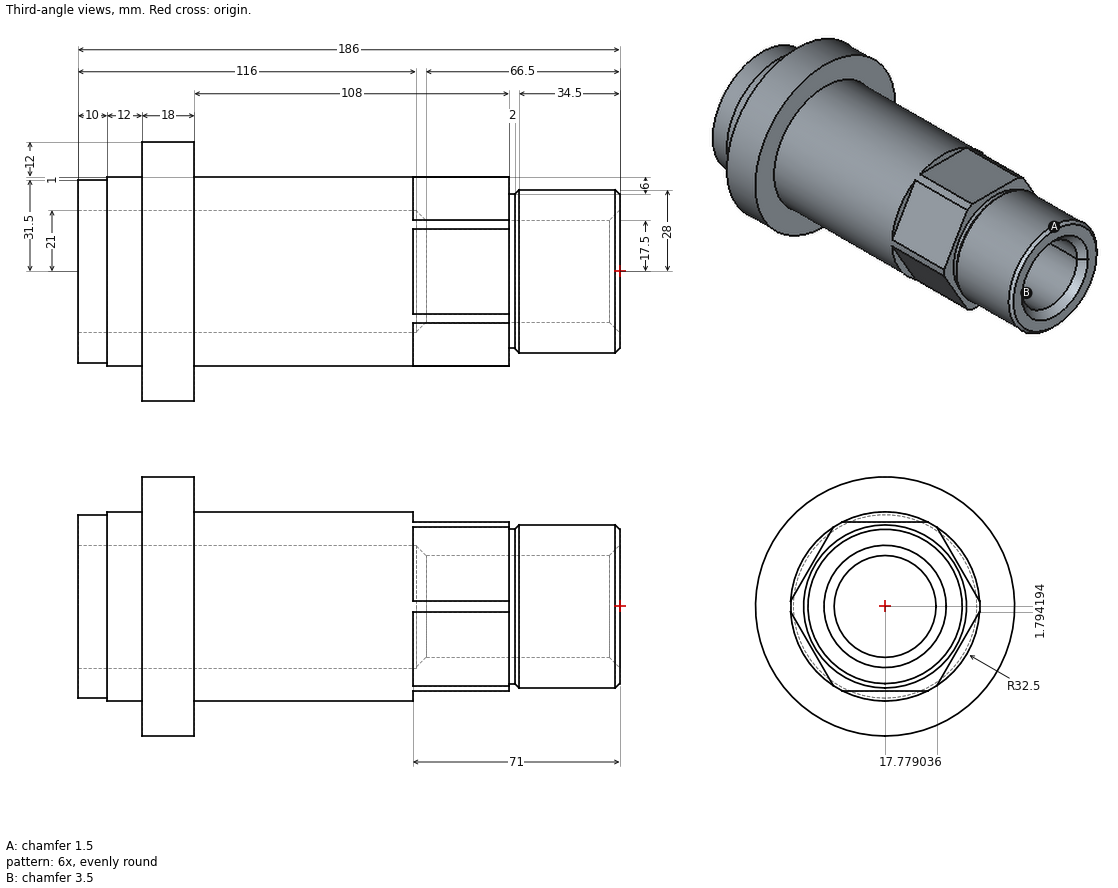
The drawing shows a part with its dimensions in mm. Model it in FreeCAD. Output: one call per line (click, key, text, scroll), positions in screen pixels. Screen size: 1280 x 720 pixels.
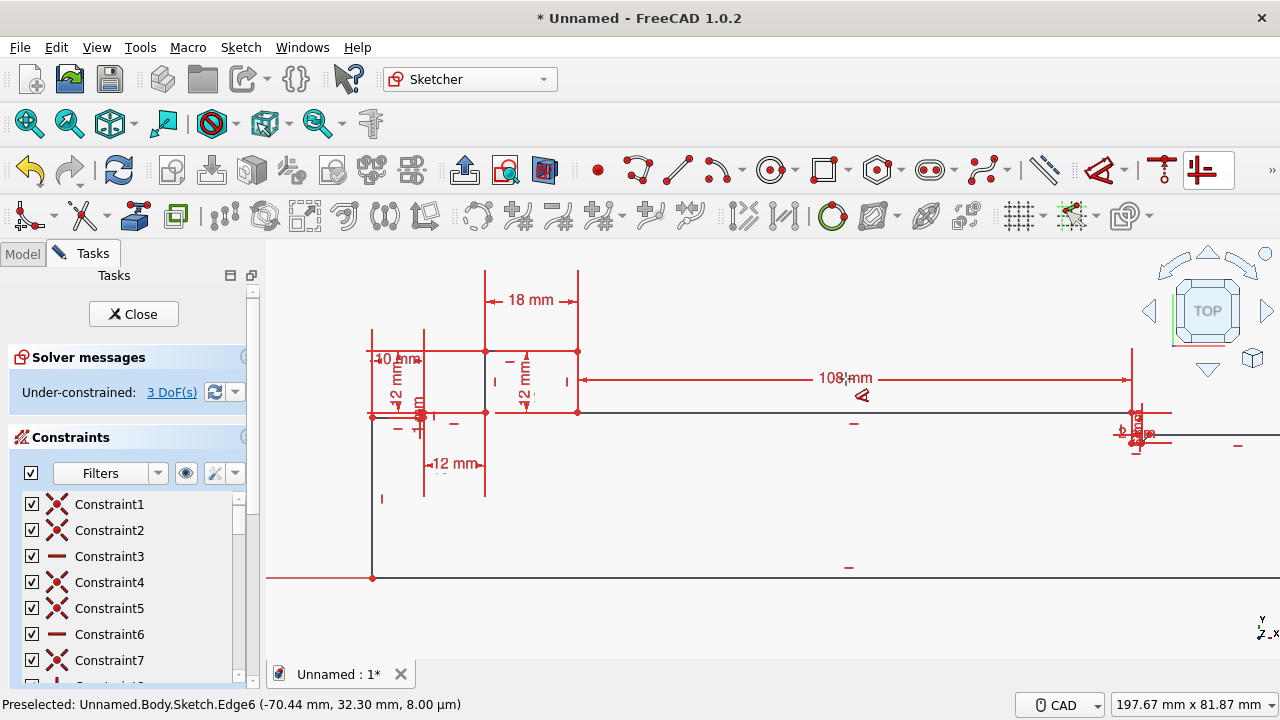
click(659, 578)
click(744, 612)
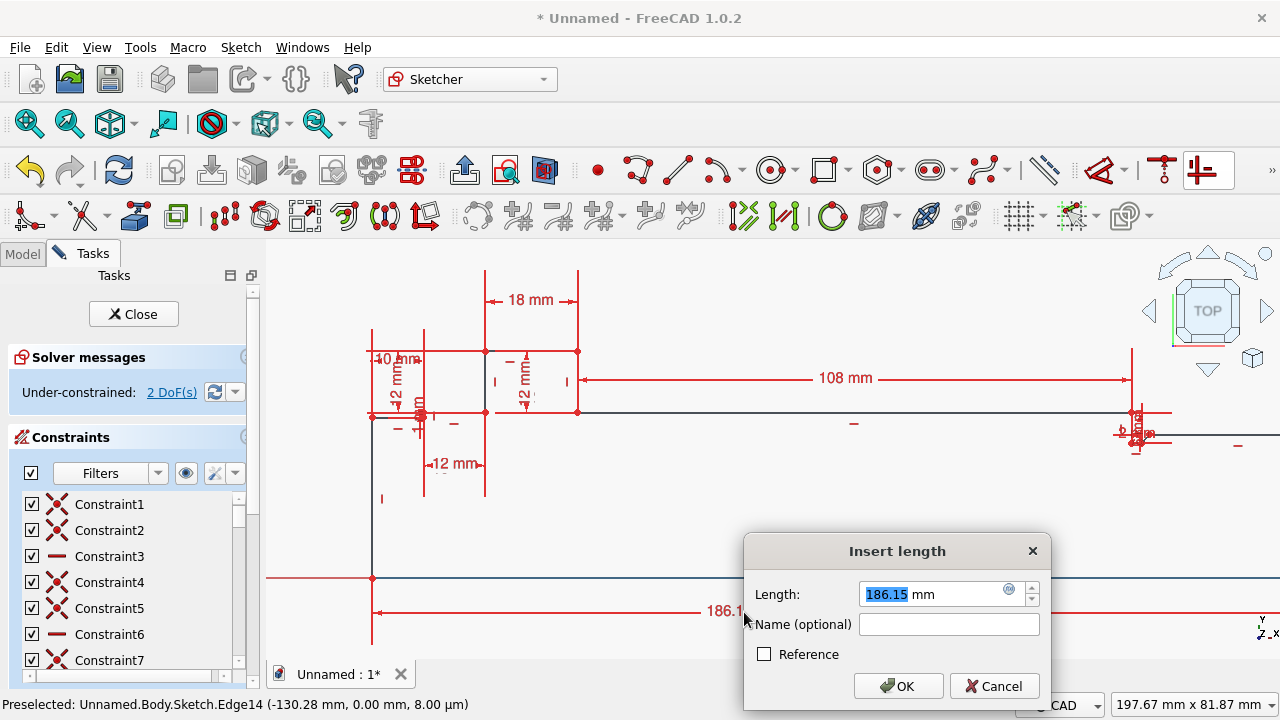
text(186)
key(Return)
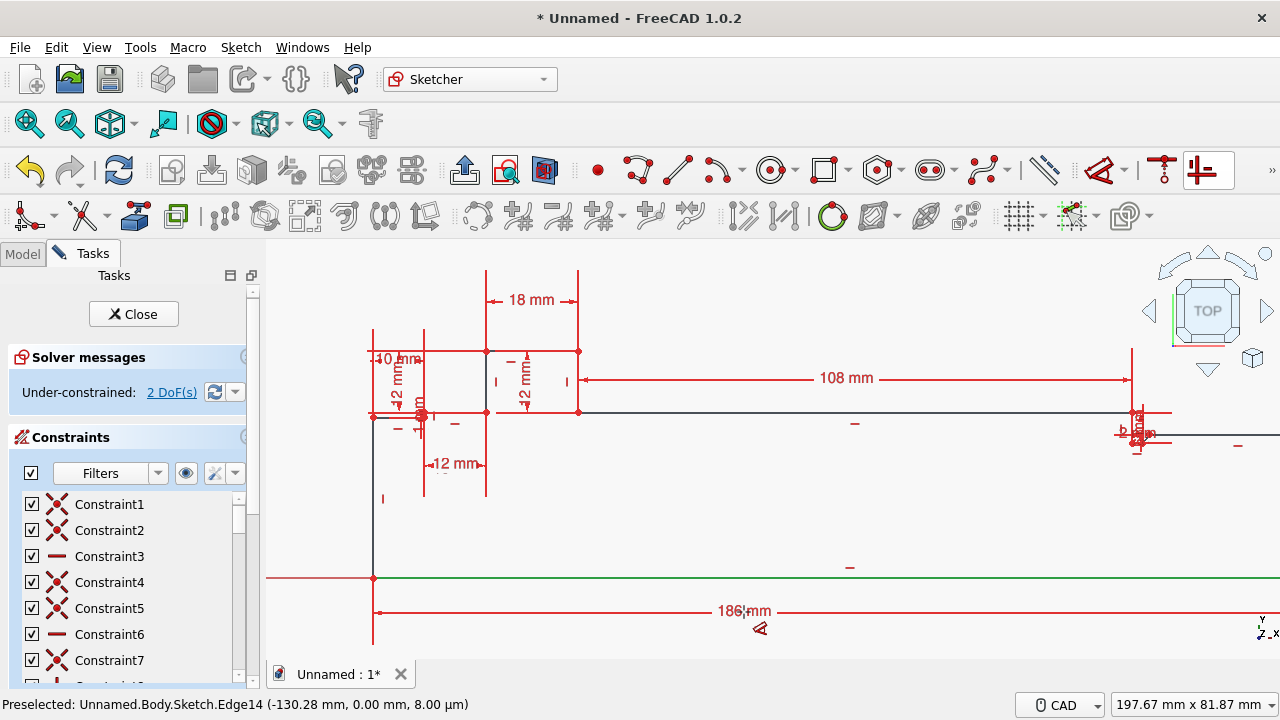
scroll(408, 418, down, 2)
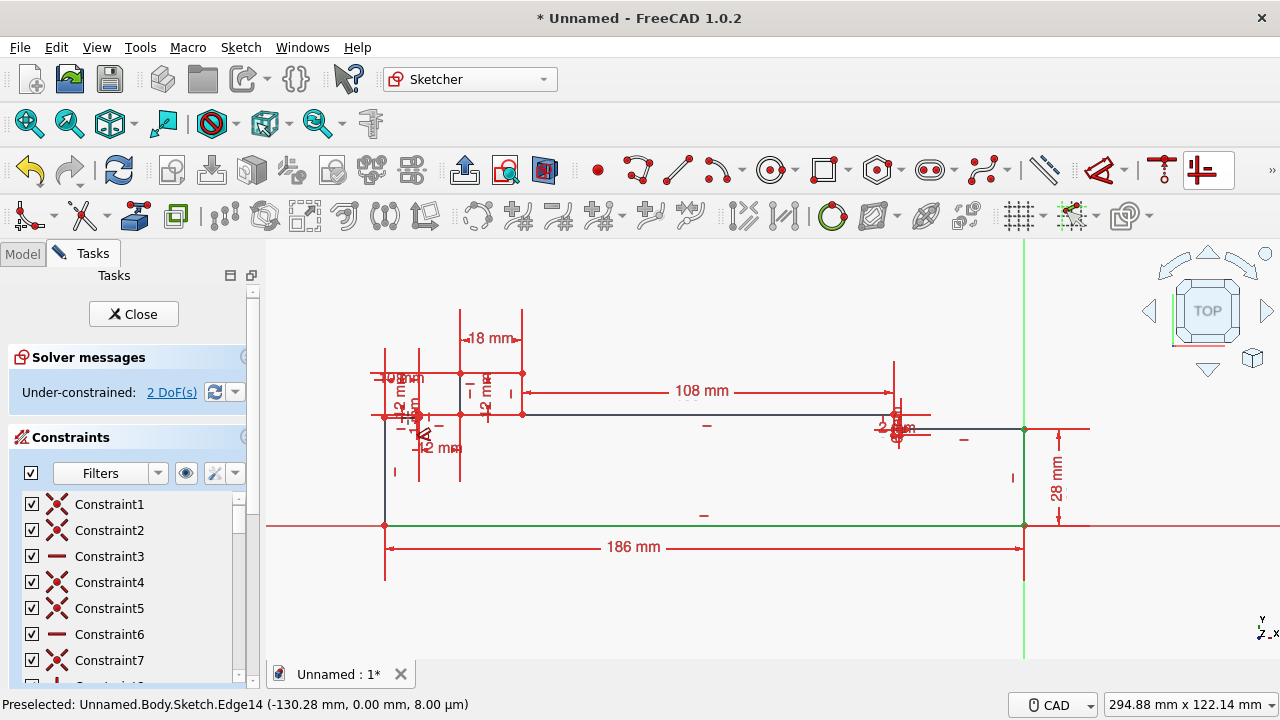
click(989, 429)
click(965, 395)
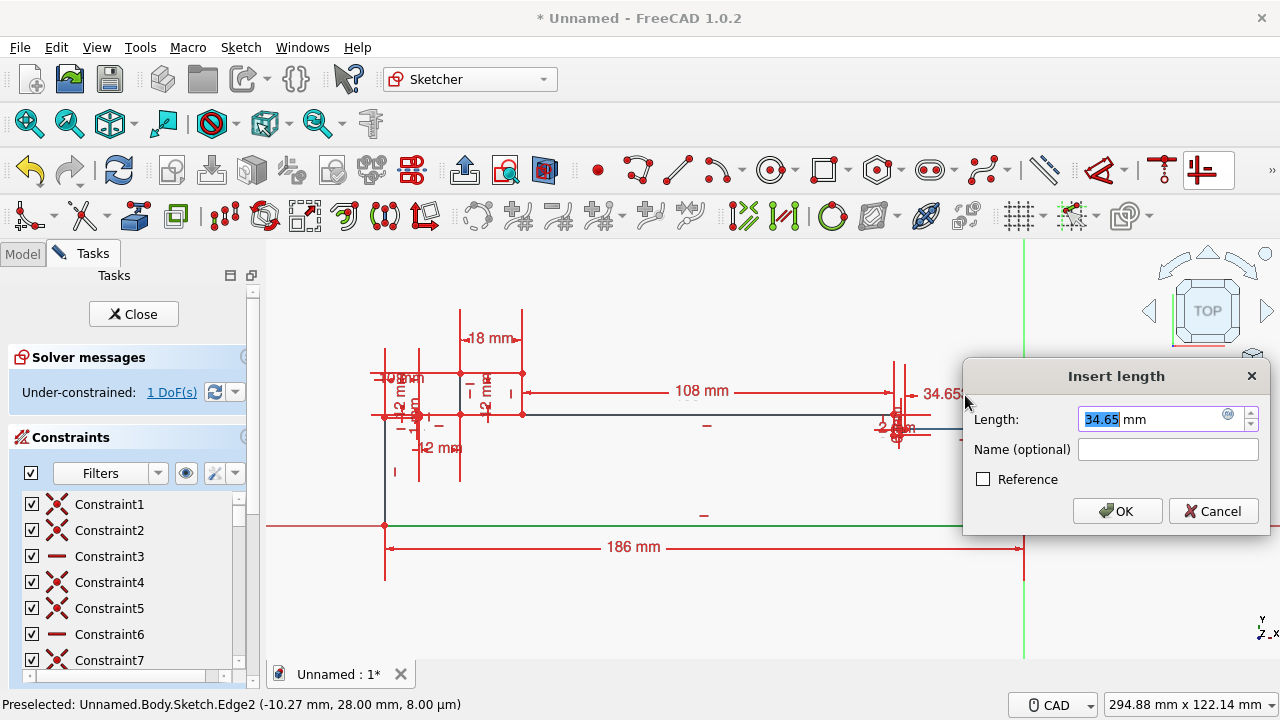
text(34.5)
key(Return)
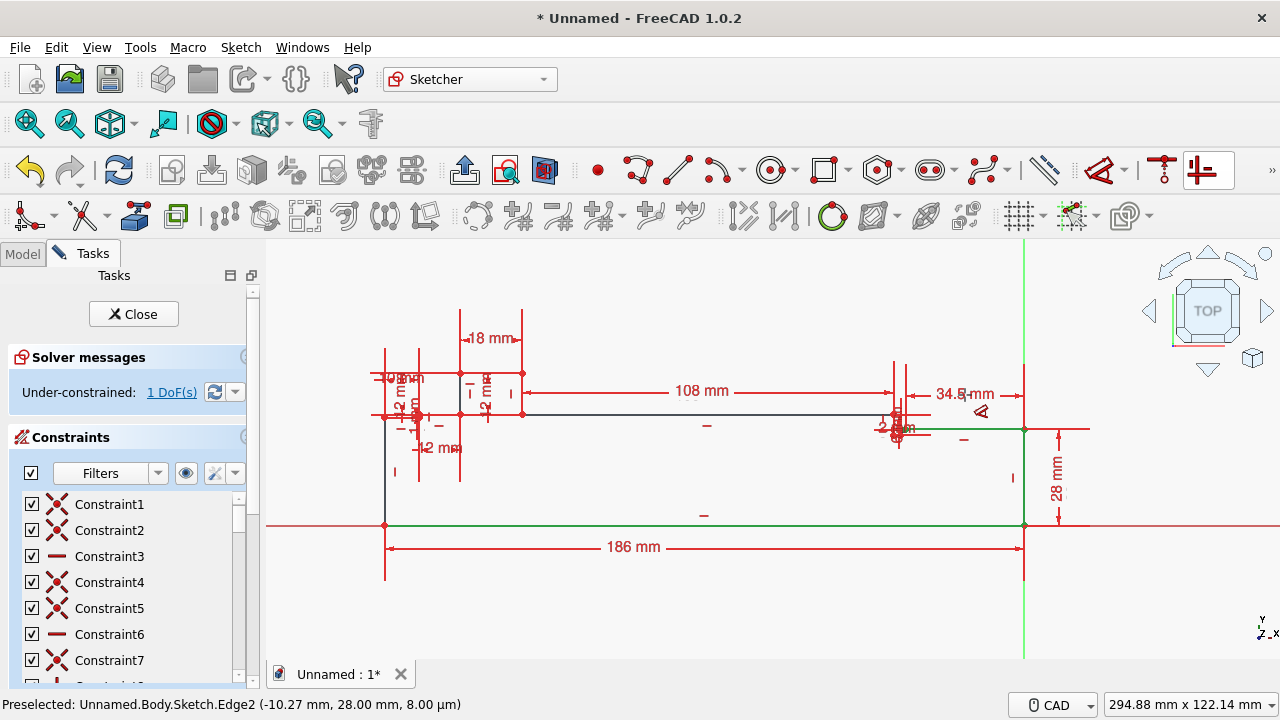
click(385, 450)
click(351, 472)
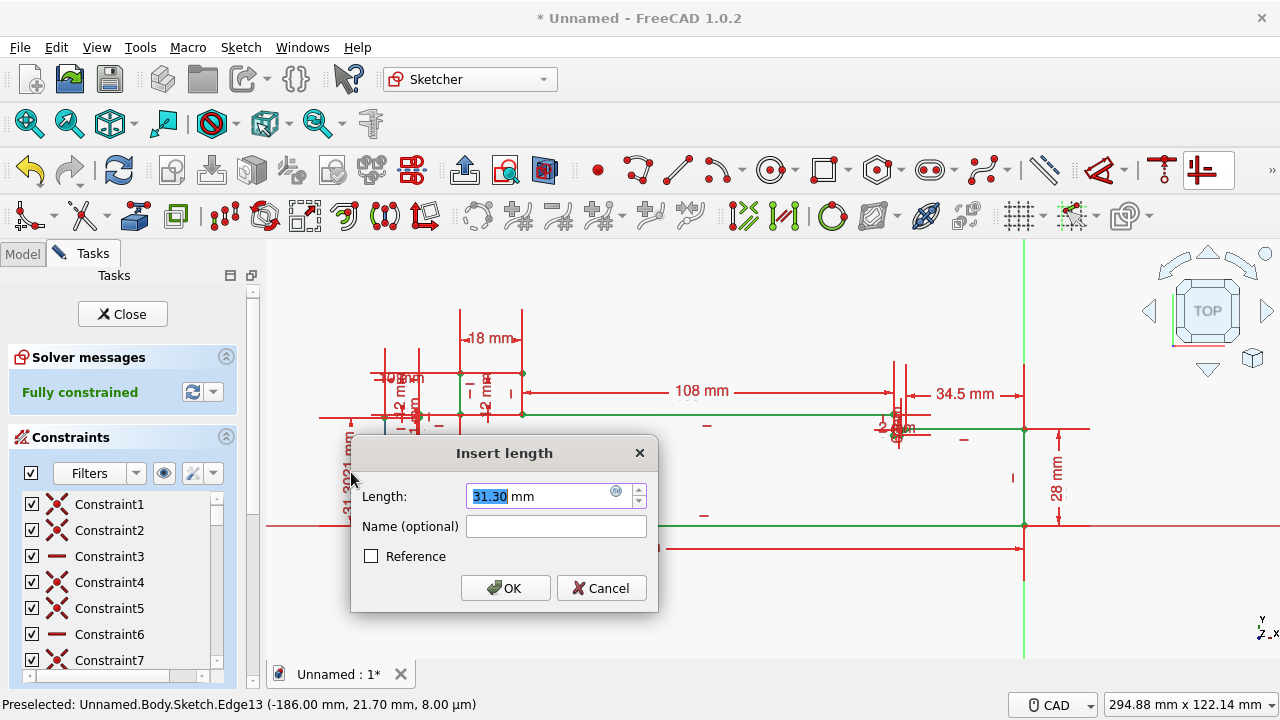
text(31.5)
key(Return)
key(Escape)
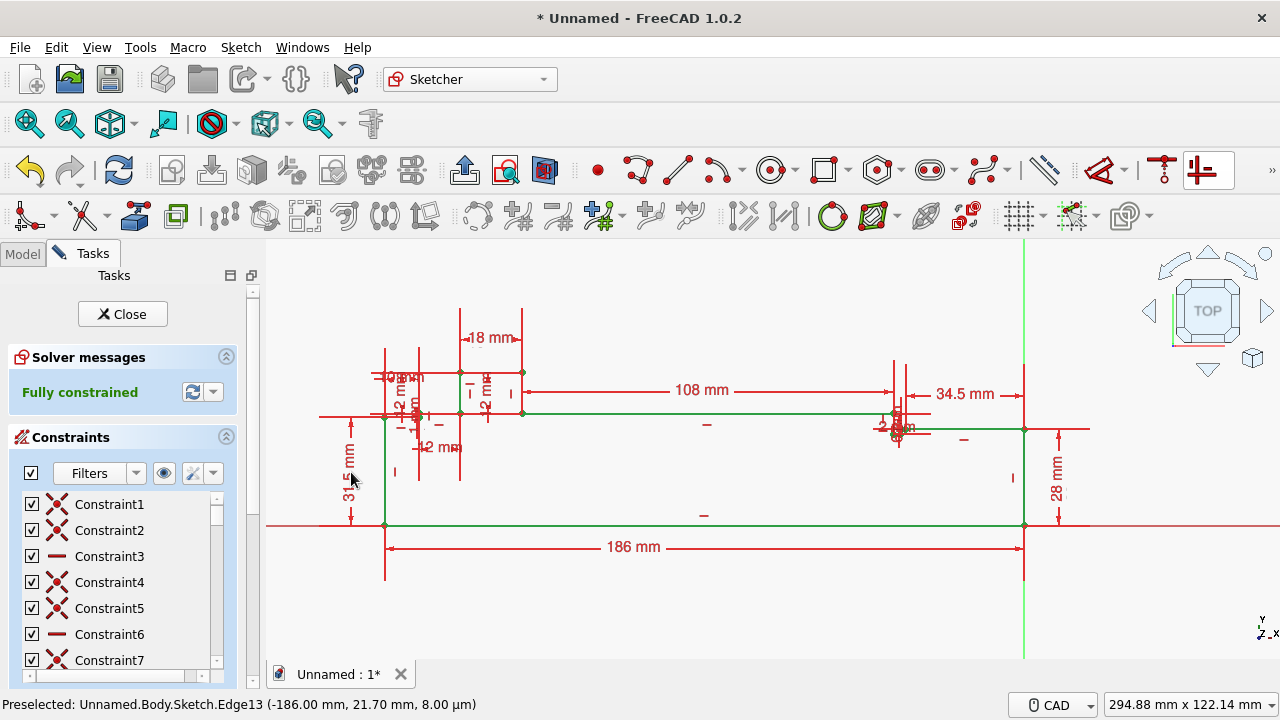
click(123, 314)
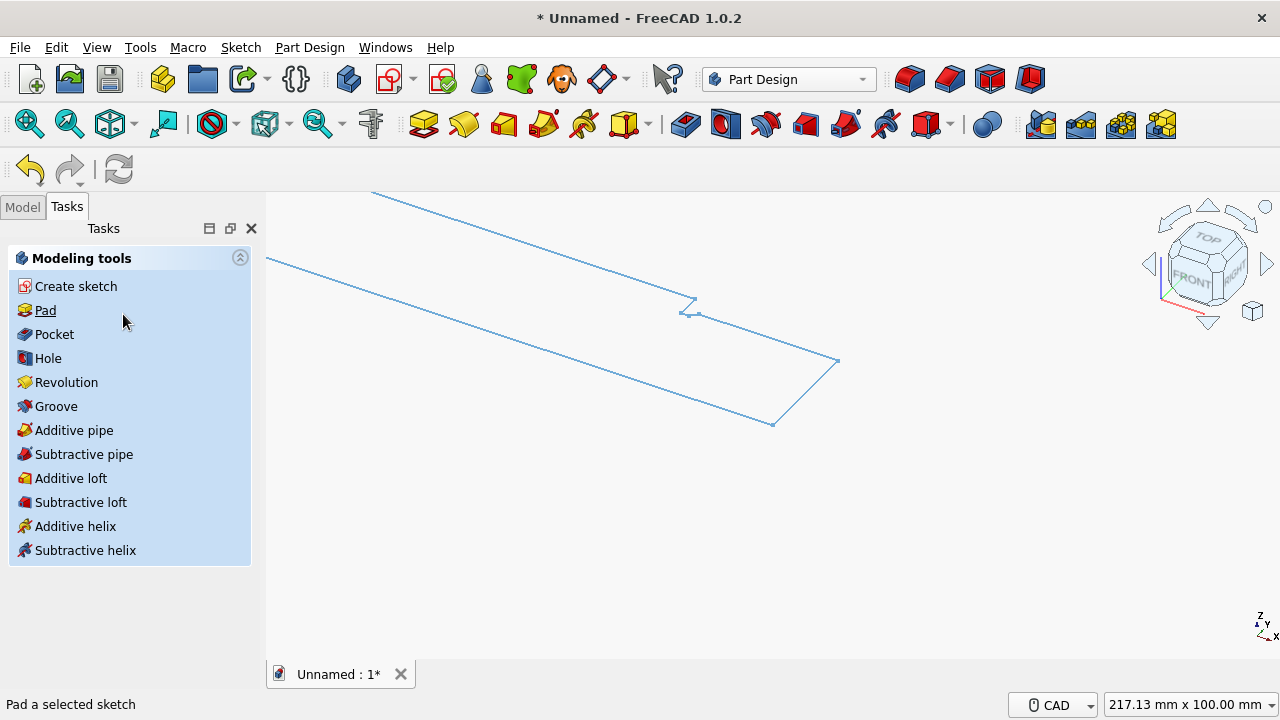
click(464, 124)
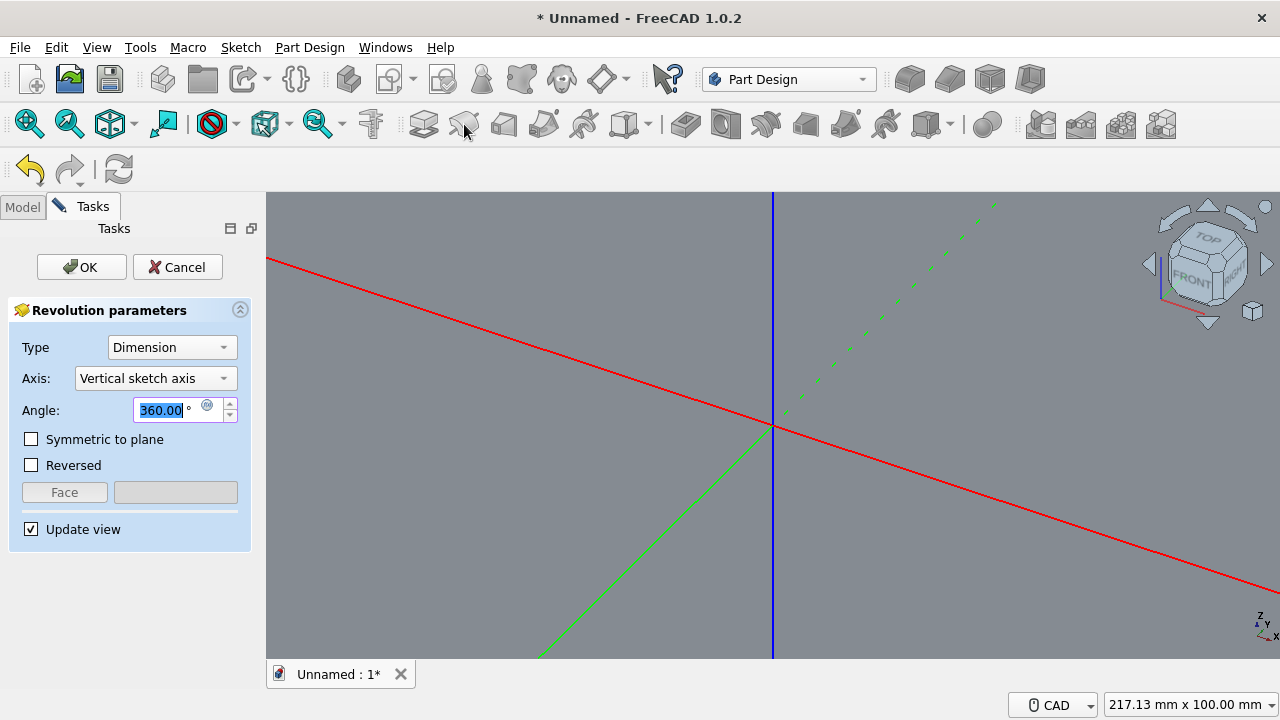
click(156, 378)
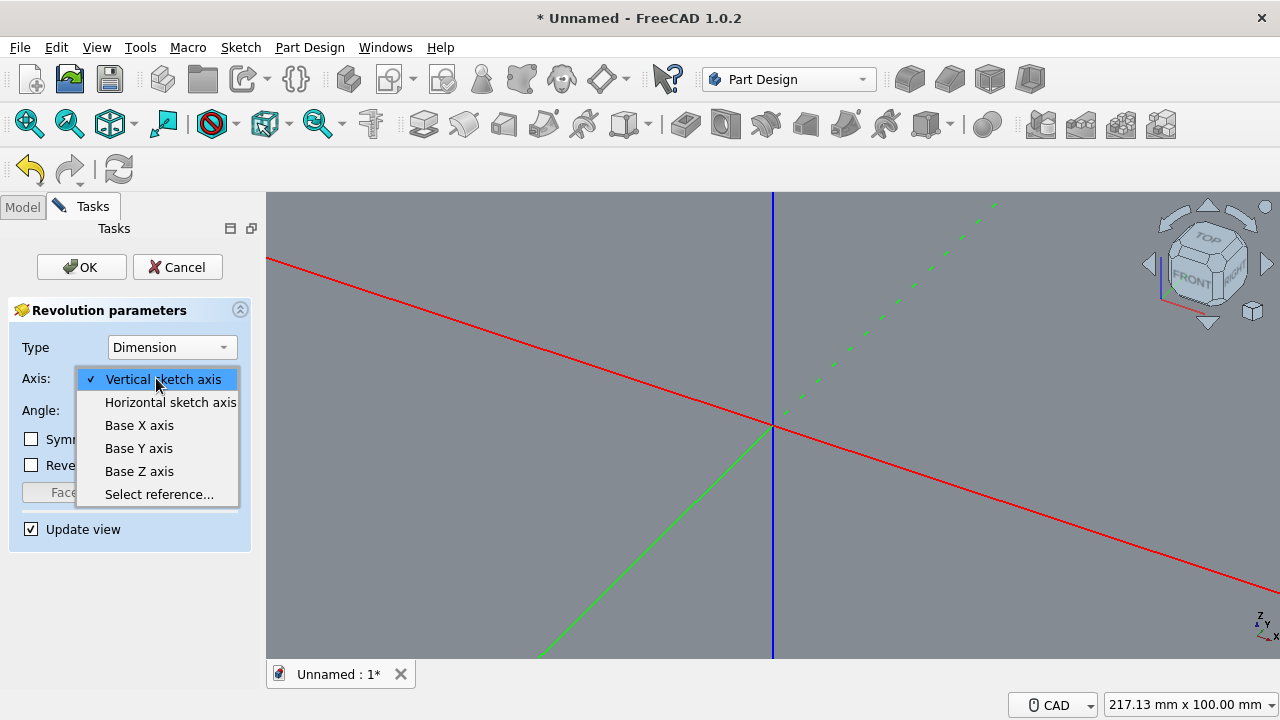
click(156, 402)